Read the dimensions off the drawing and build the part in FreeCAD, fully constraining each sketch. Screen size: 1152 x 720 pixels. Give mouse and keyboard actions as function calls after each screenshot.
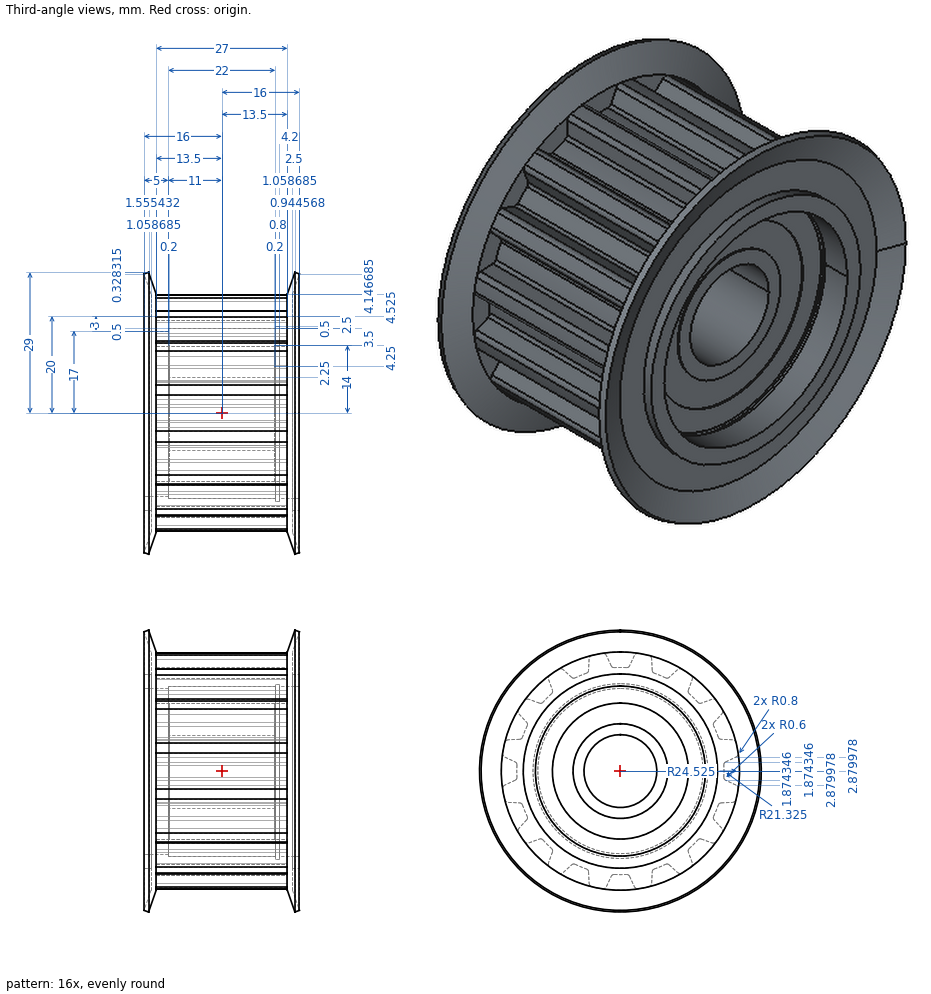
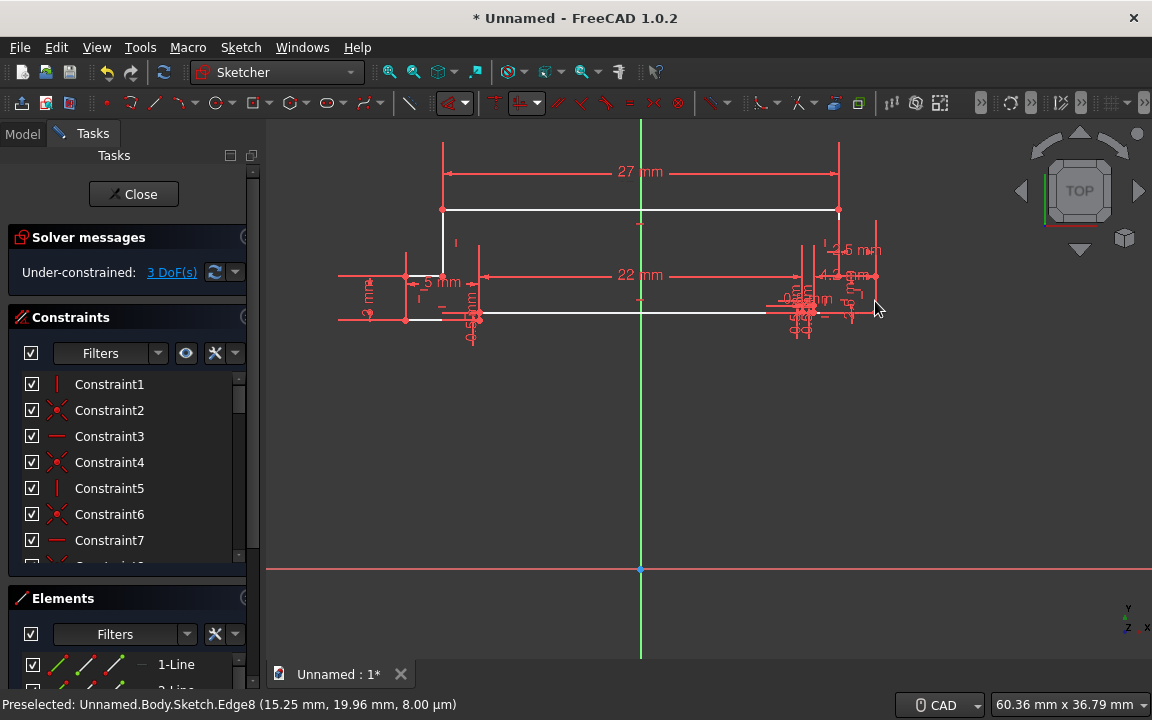
scroll(479, 320, up, 3)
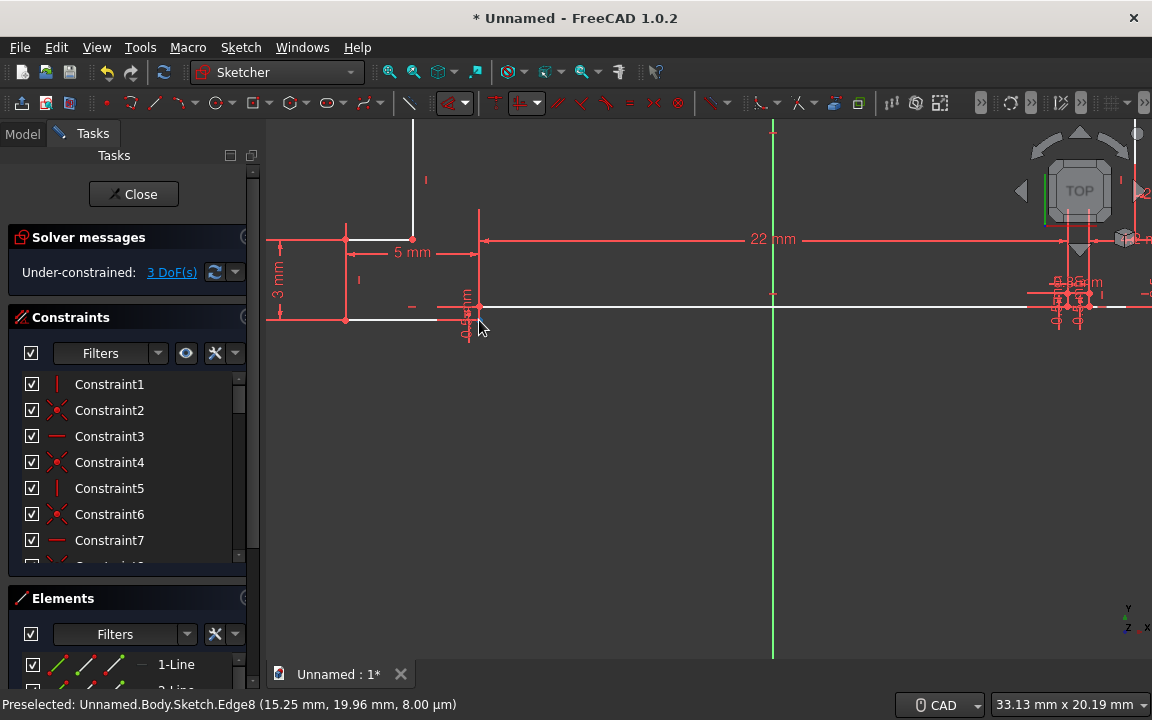
click(479, 320)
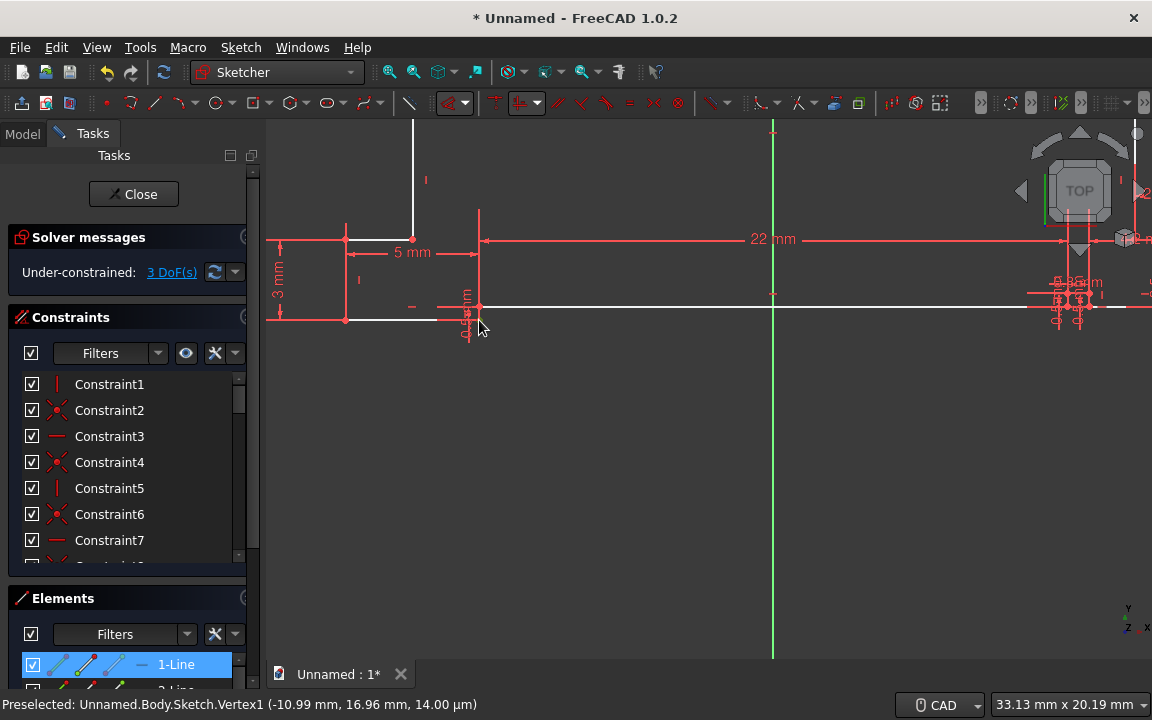
click(468, 104)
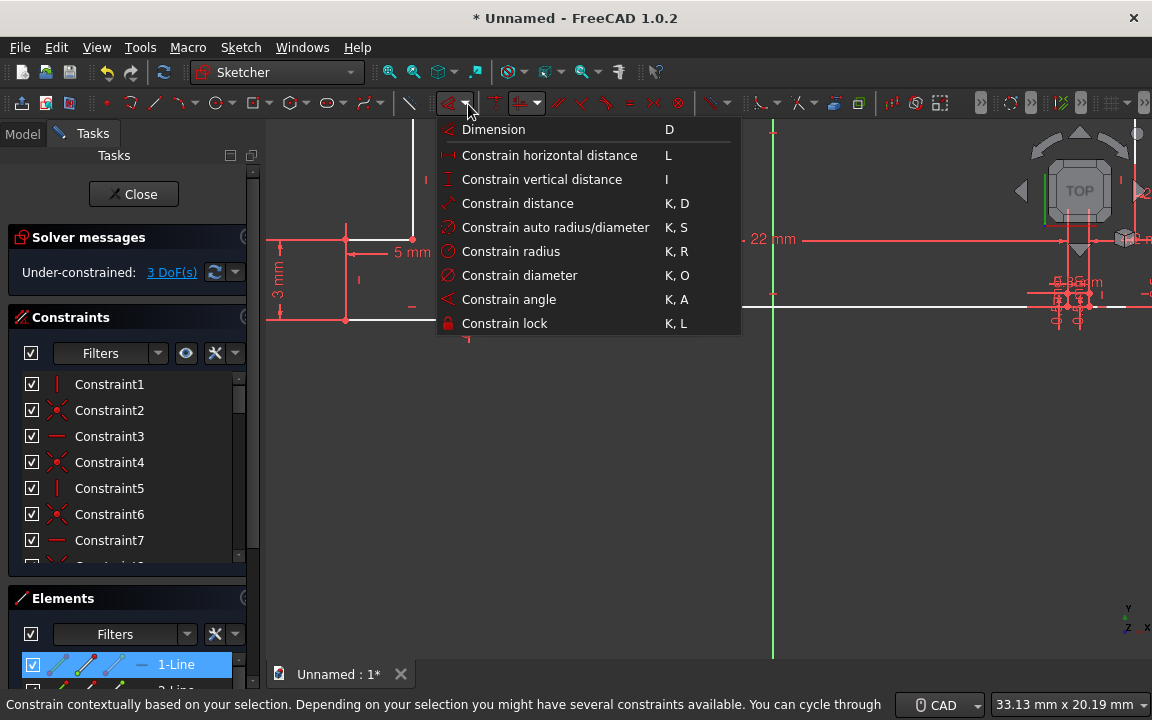
click(589, 155)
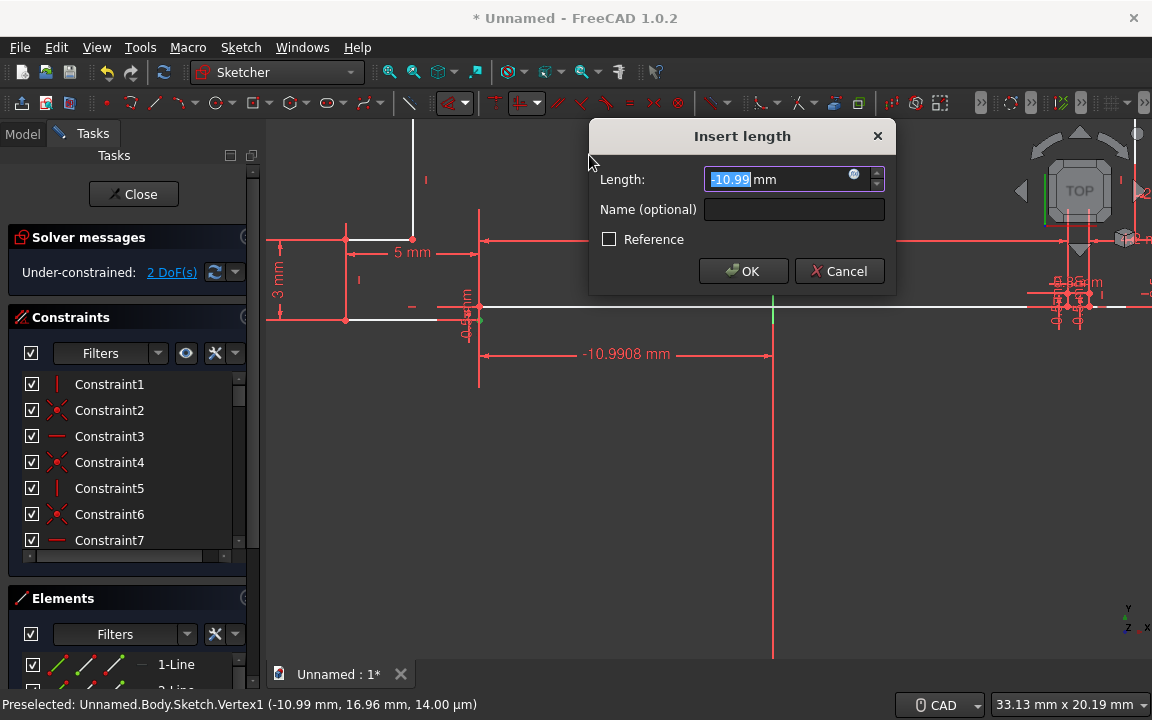
text(-11)
key(Return)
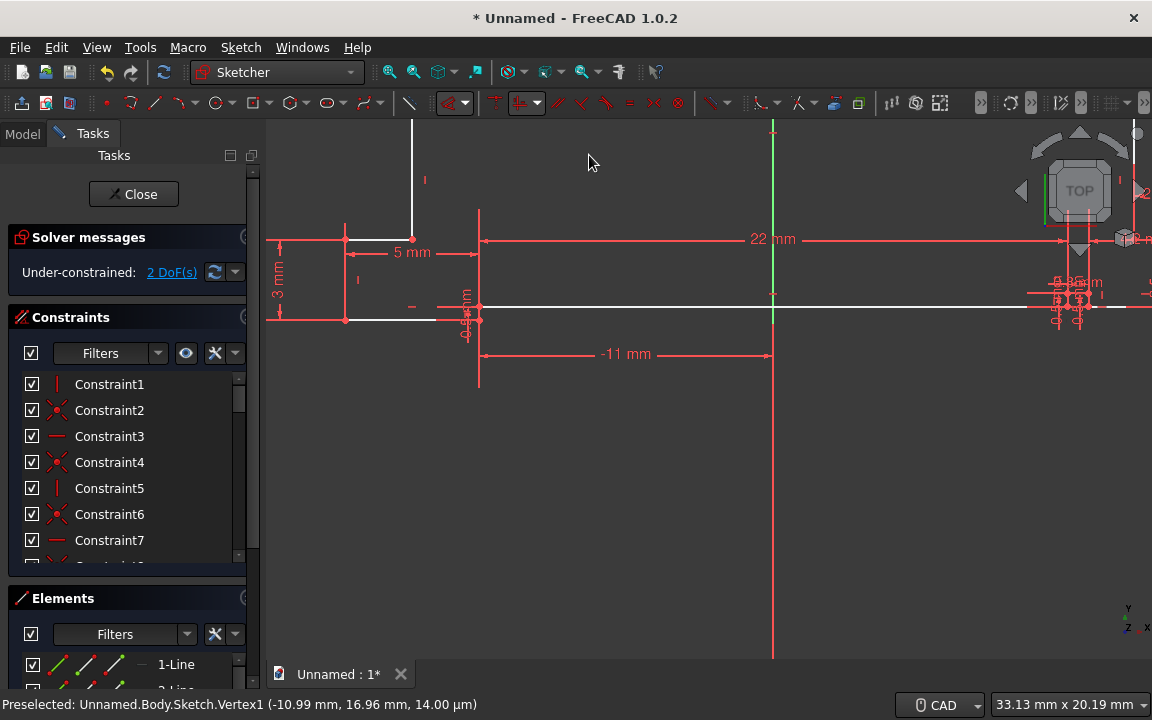
click(479, 320)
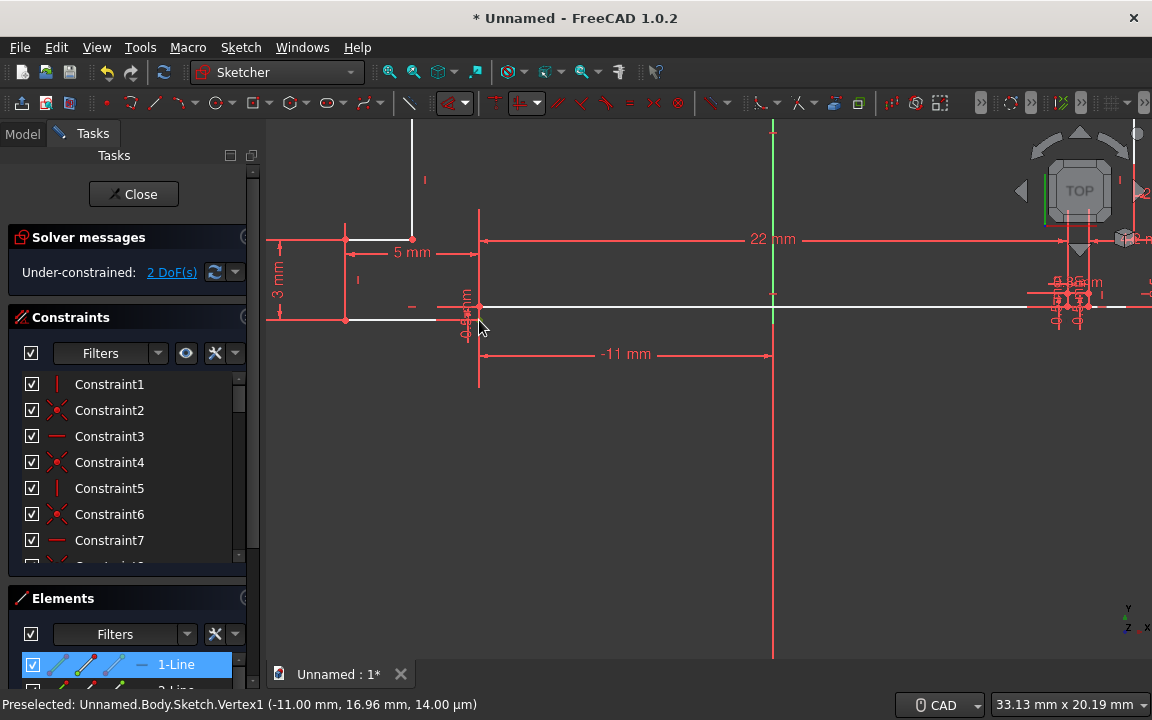
click(468, 104)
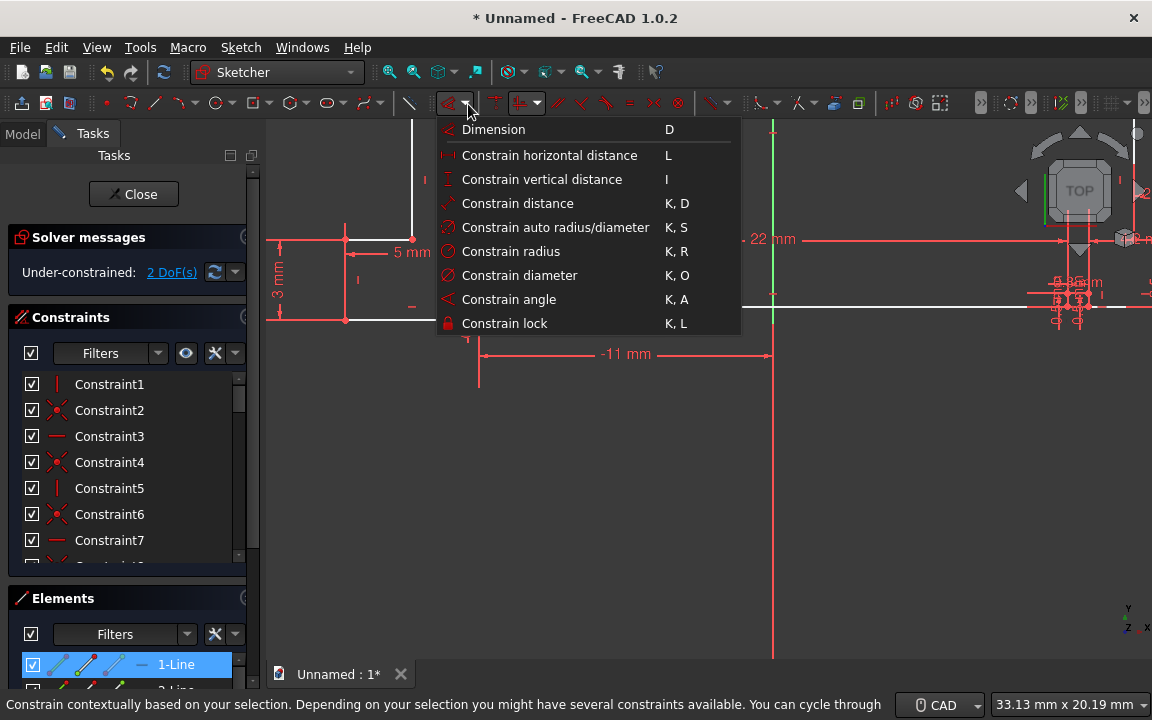
click(589, 179)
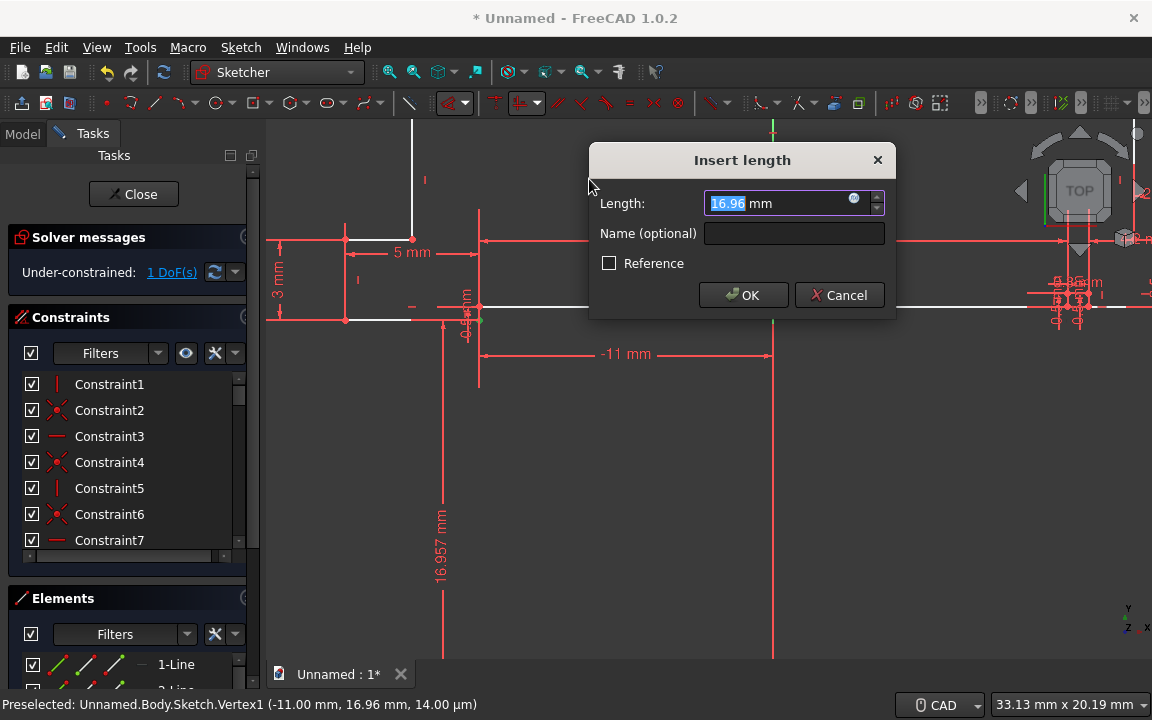
text(17)
key(Return)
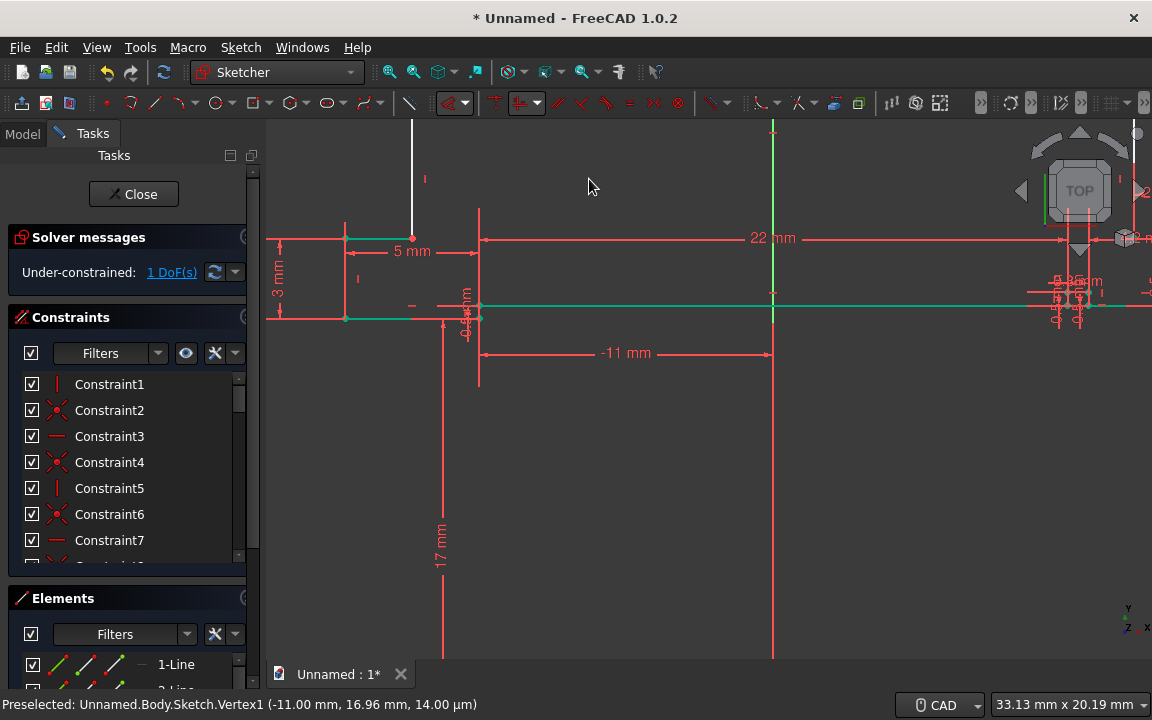
scroll(479, 320, down, 3)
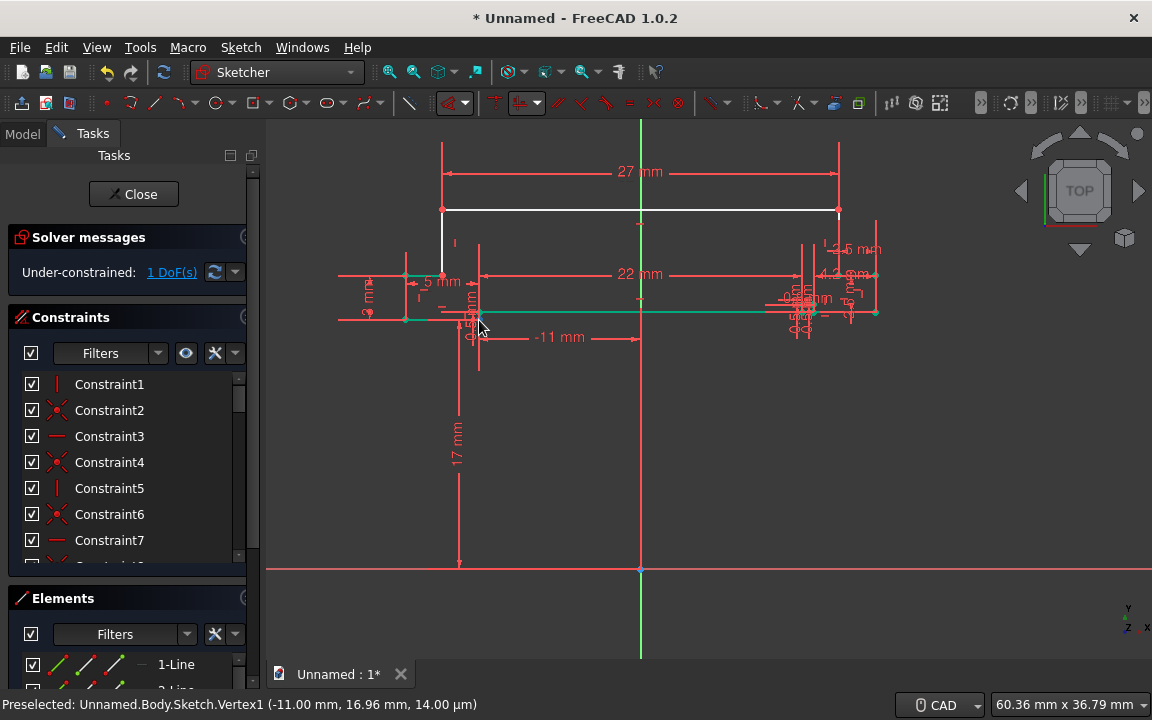
click(839, 229)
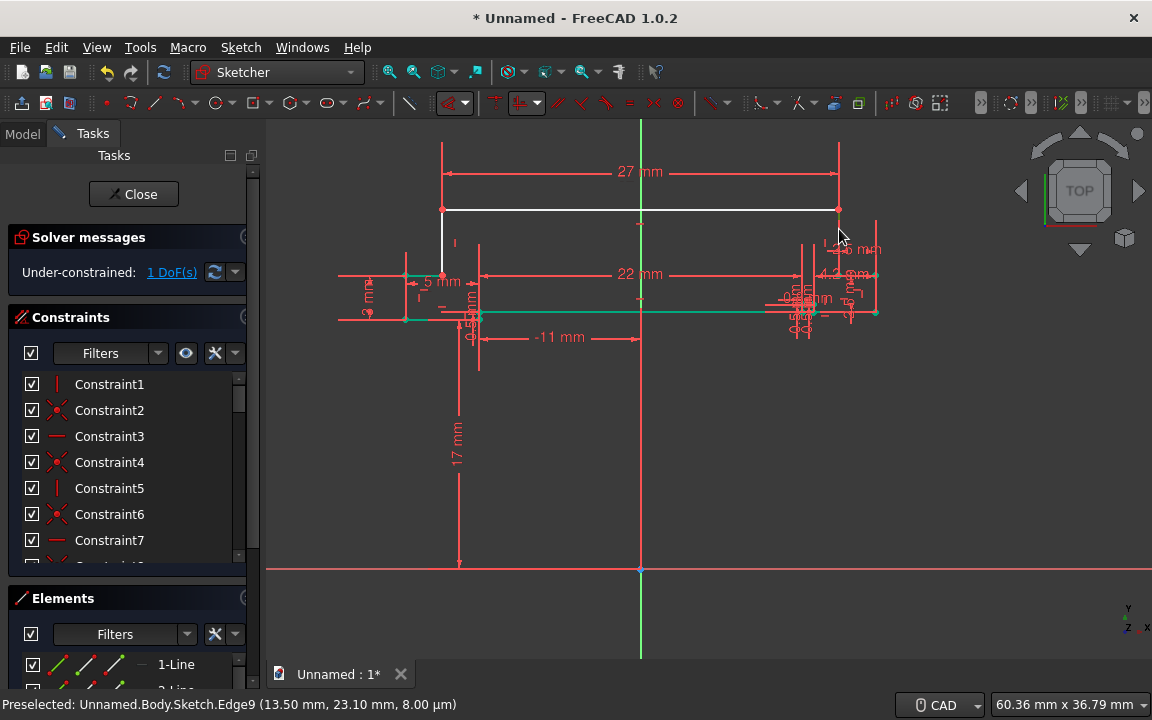
click(468, 104)